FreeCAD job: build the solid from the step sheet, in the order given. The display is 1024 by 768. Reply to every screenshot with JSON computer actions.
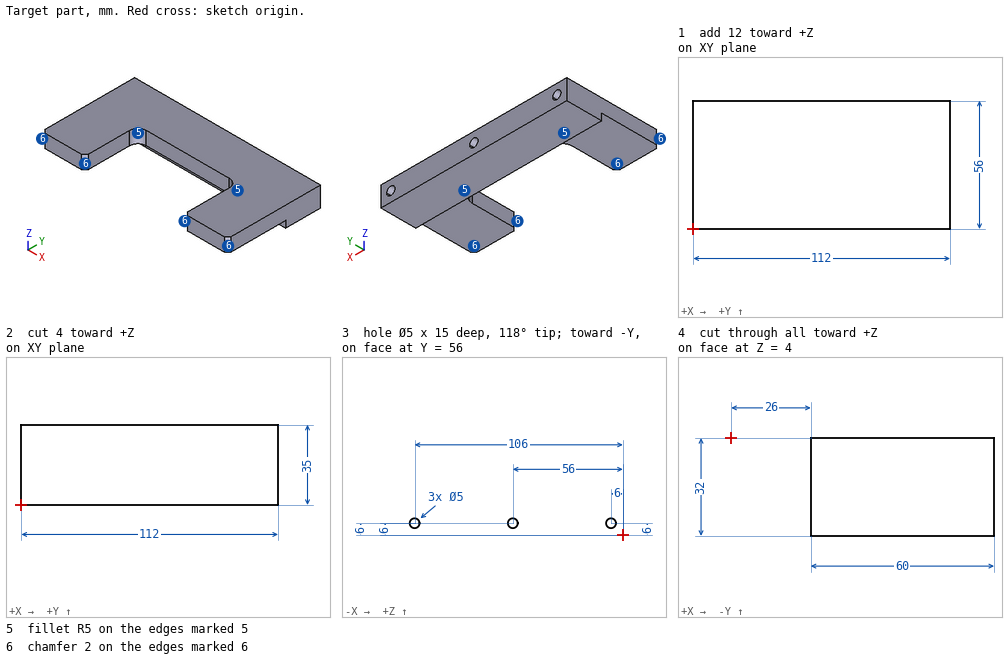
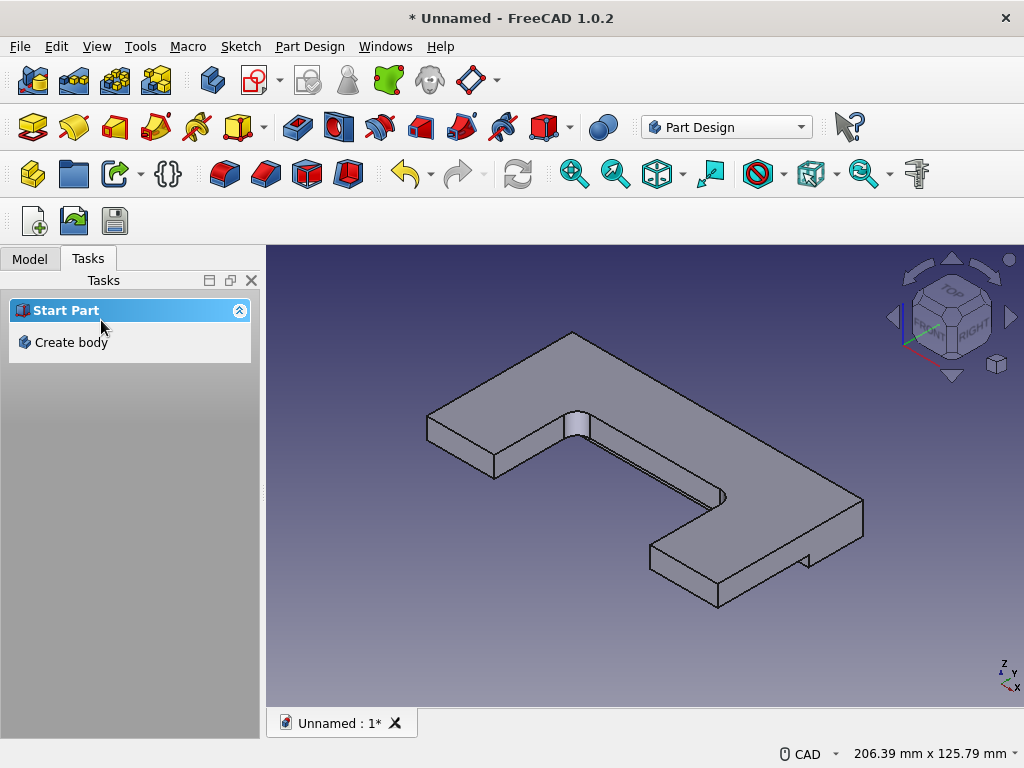
{"action": "left_click", "coordinate": [494, 466]}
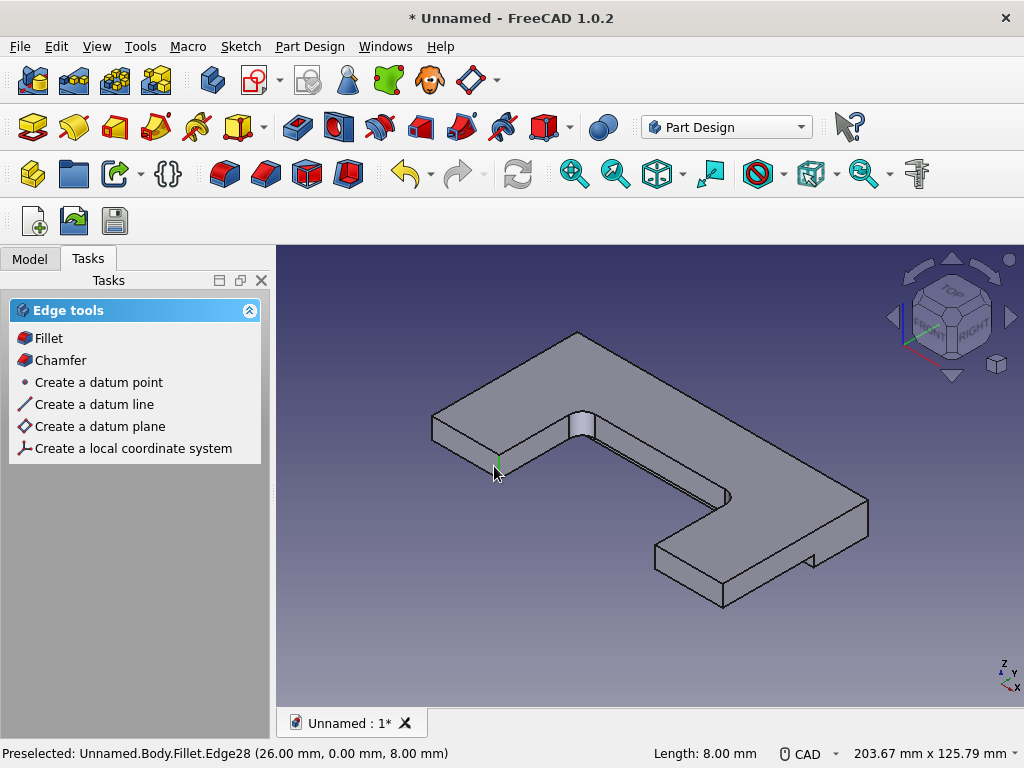
{"action": "left_click", "coordinate": [723, 595], "text": "ctrl"}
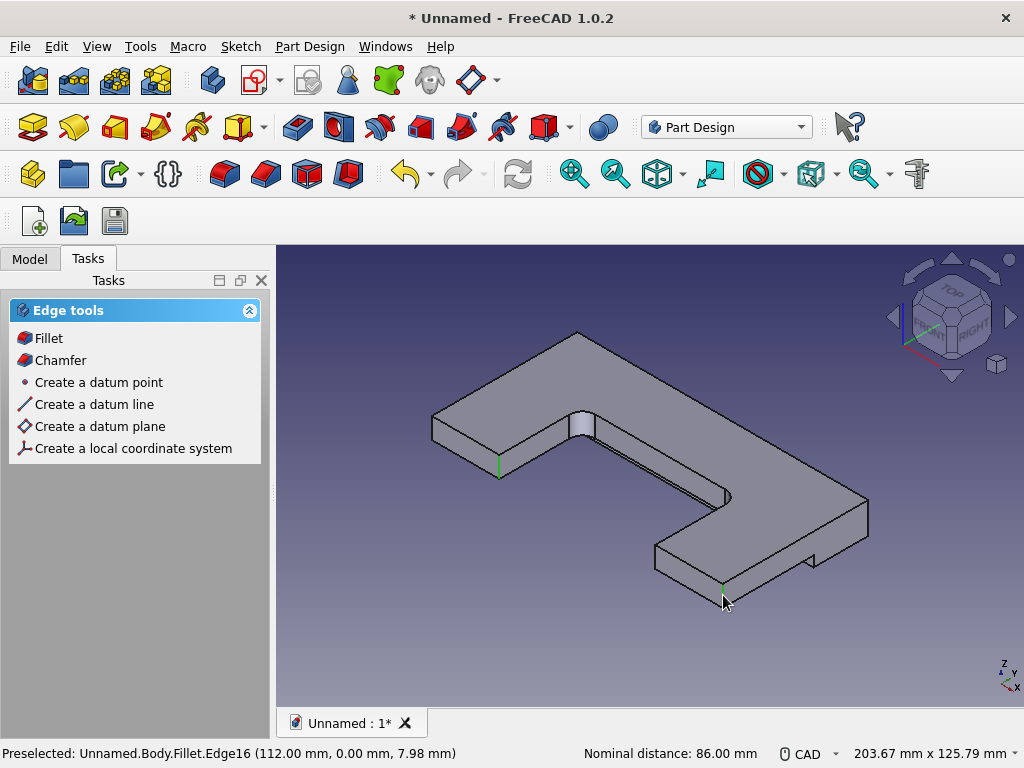
{"action": "key", "text": "2"}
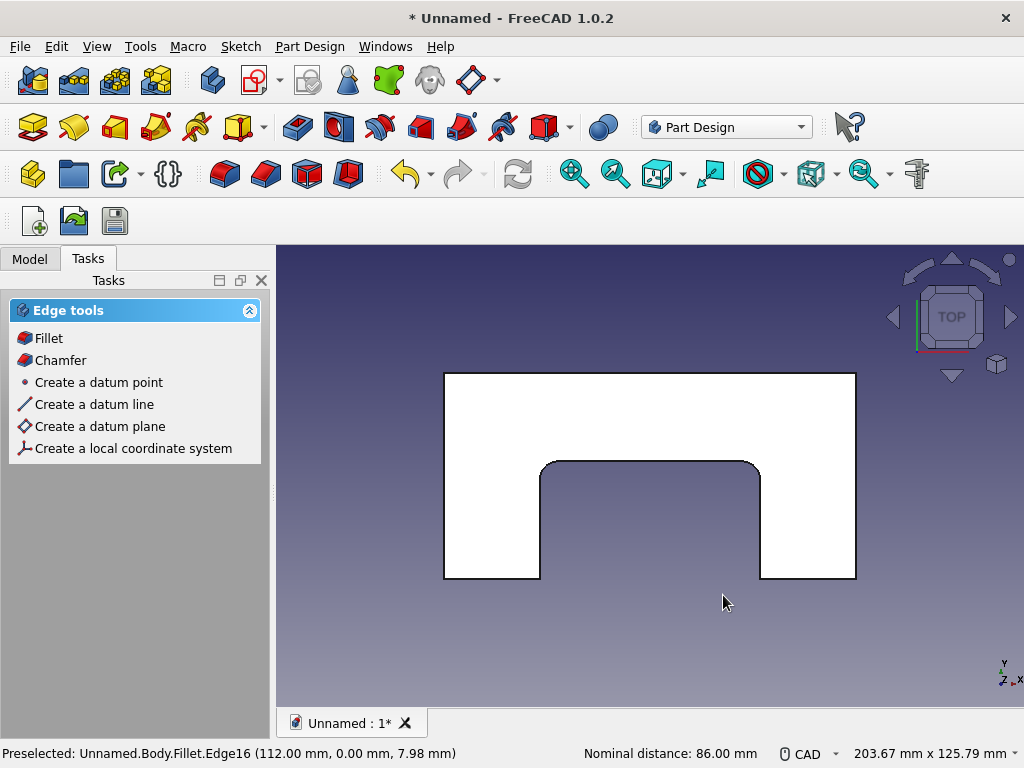
{"action": "key", "text": "0"}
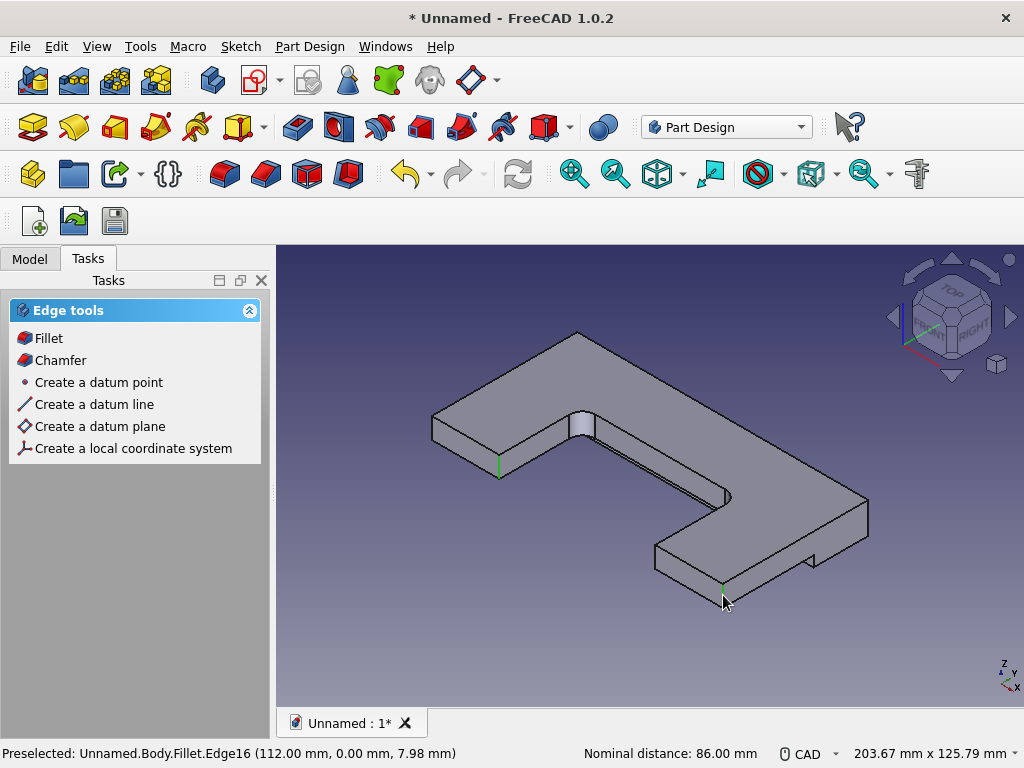
{"action": "key", "text": "1"}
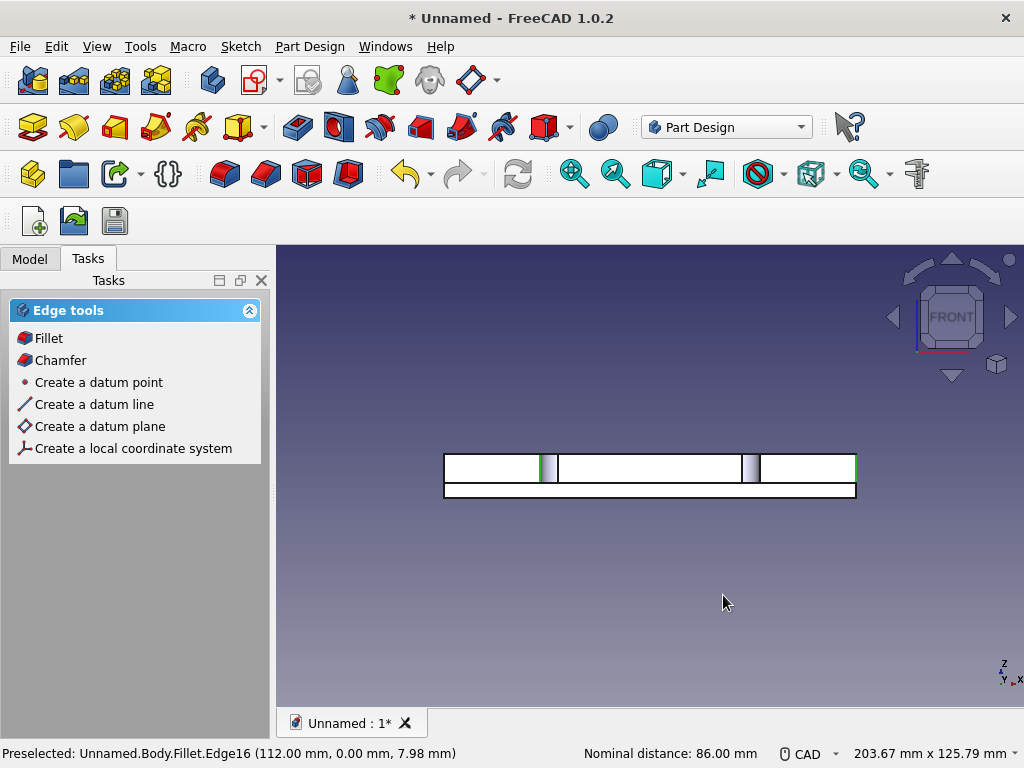
{"action": "left_click", "coordinate": [760, 468], "text": "ctrl"}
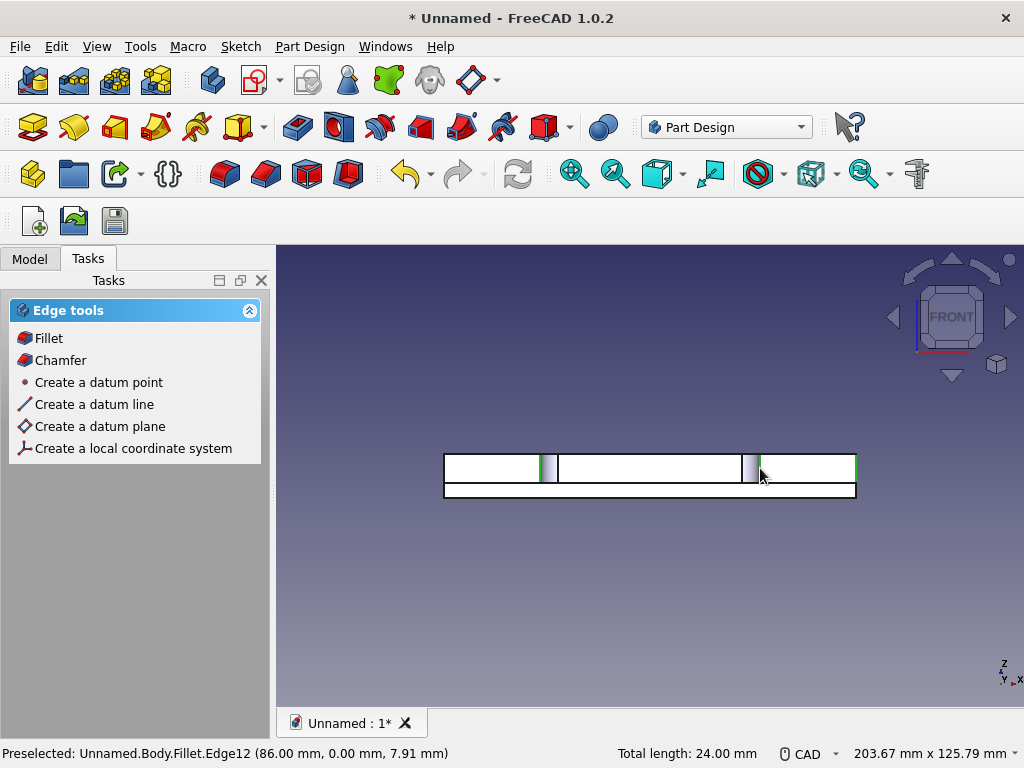
{"action": "left_click", "coordinate": [444, 468], "text": "ctrl"}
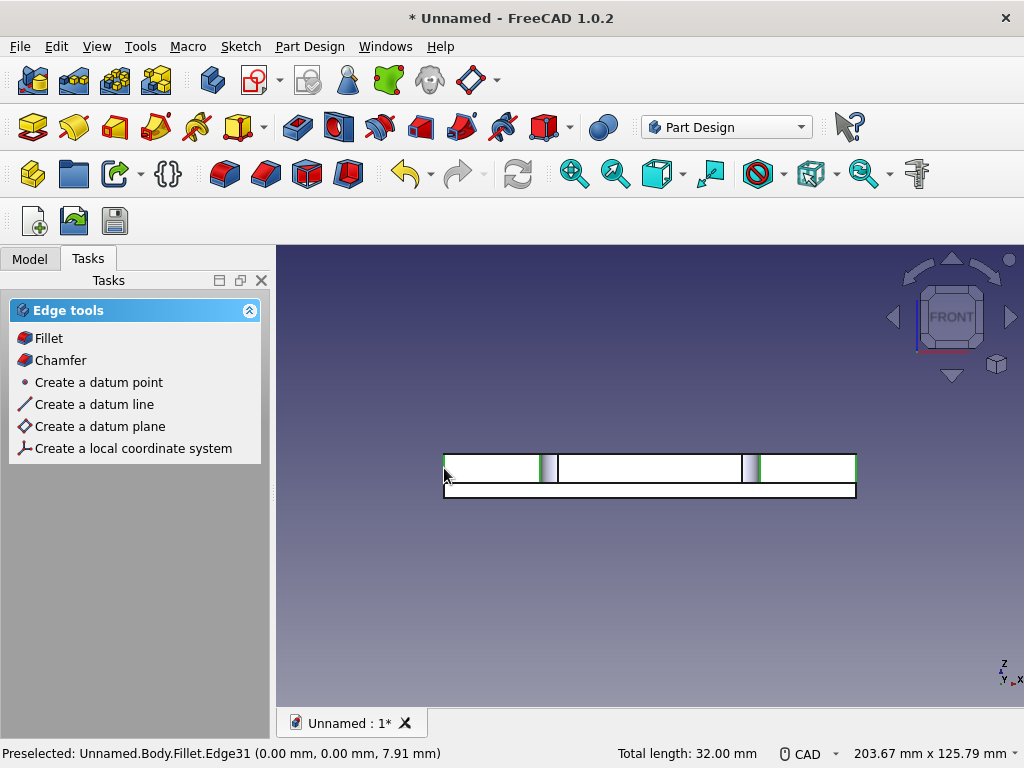
{"action": "left_click", "coordinate": [266, 174]}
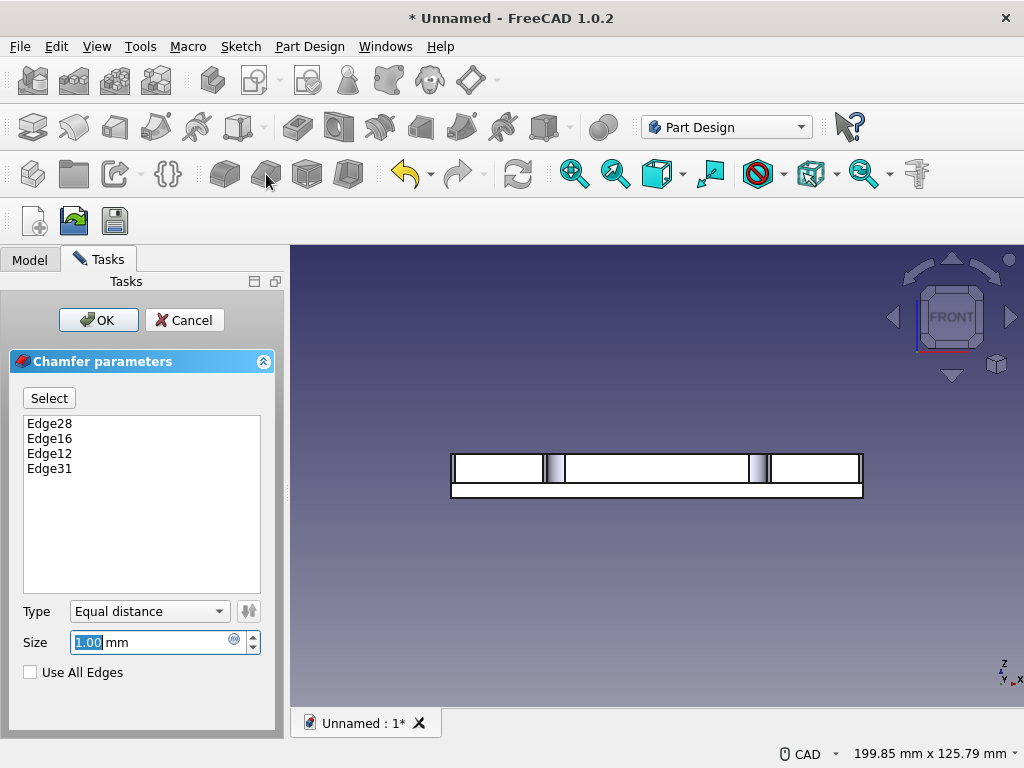
{"action": "type", "text": "2"}
{"action": "key", "text": "Tab"}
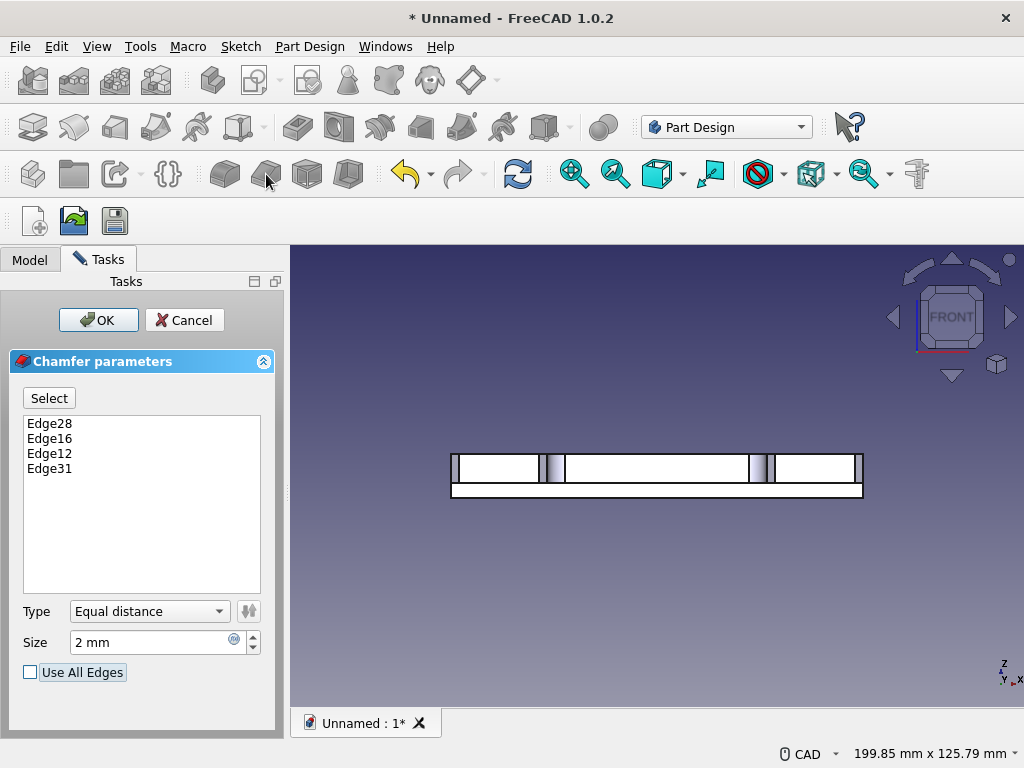
{"action": "left_click", "coordinate": [99, 320]}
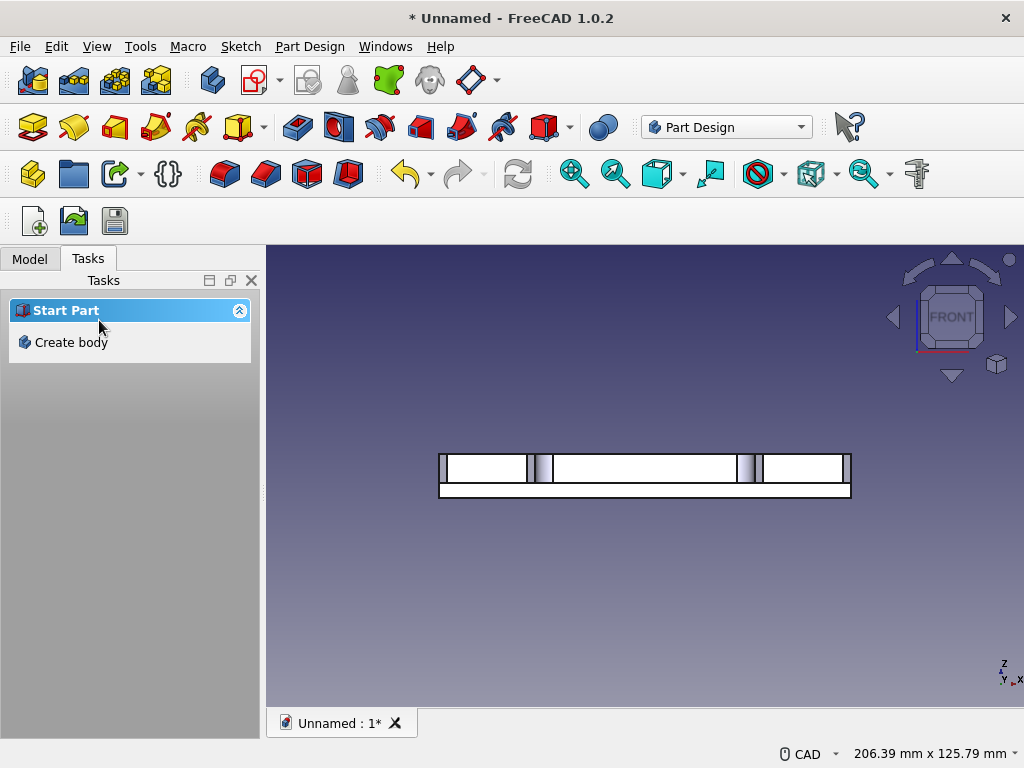
{"action": "key", "text": "0"}